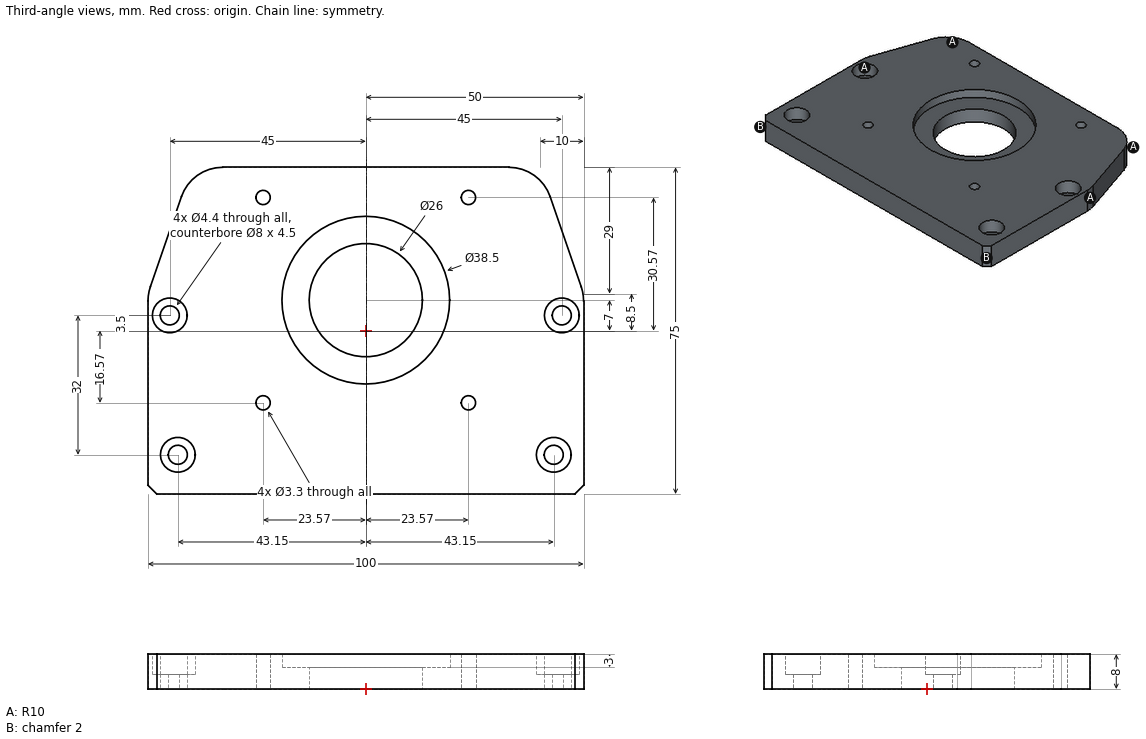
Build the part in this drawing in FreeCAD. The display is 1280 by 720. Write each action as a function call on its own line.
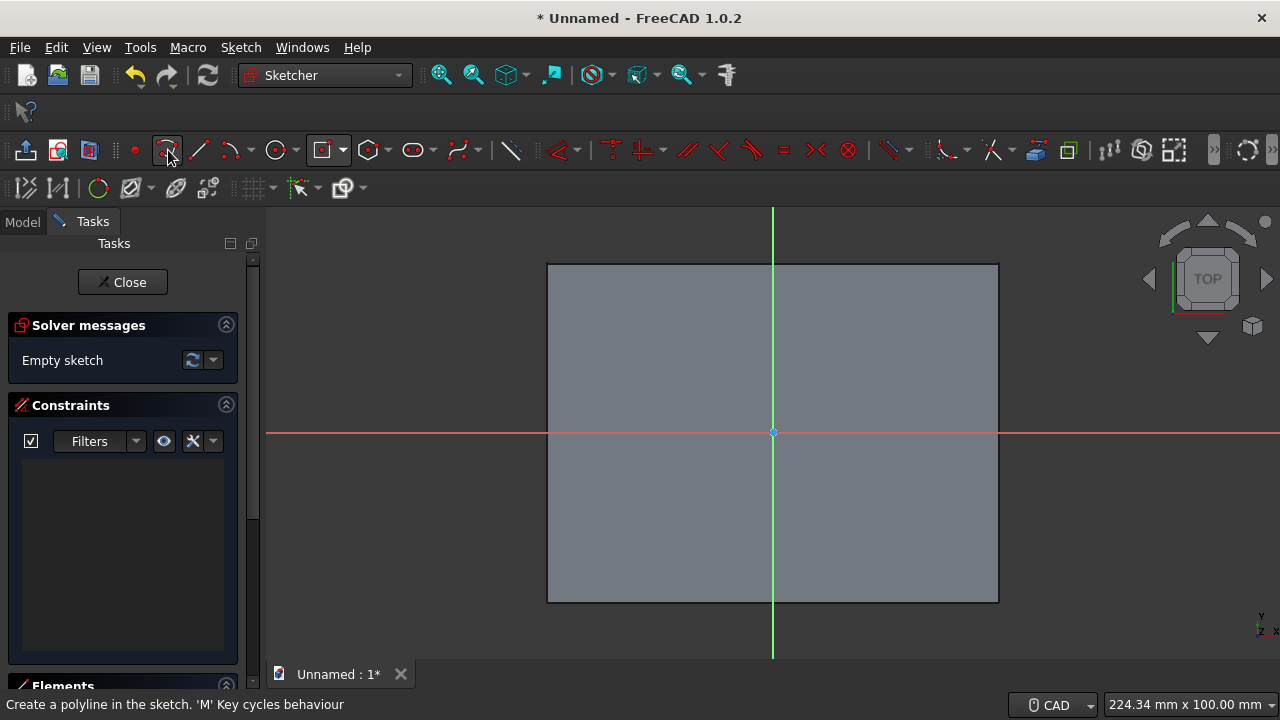
click(999, 395)
click(954, 264)
click(999, 264)
click(999, 396)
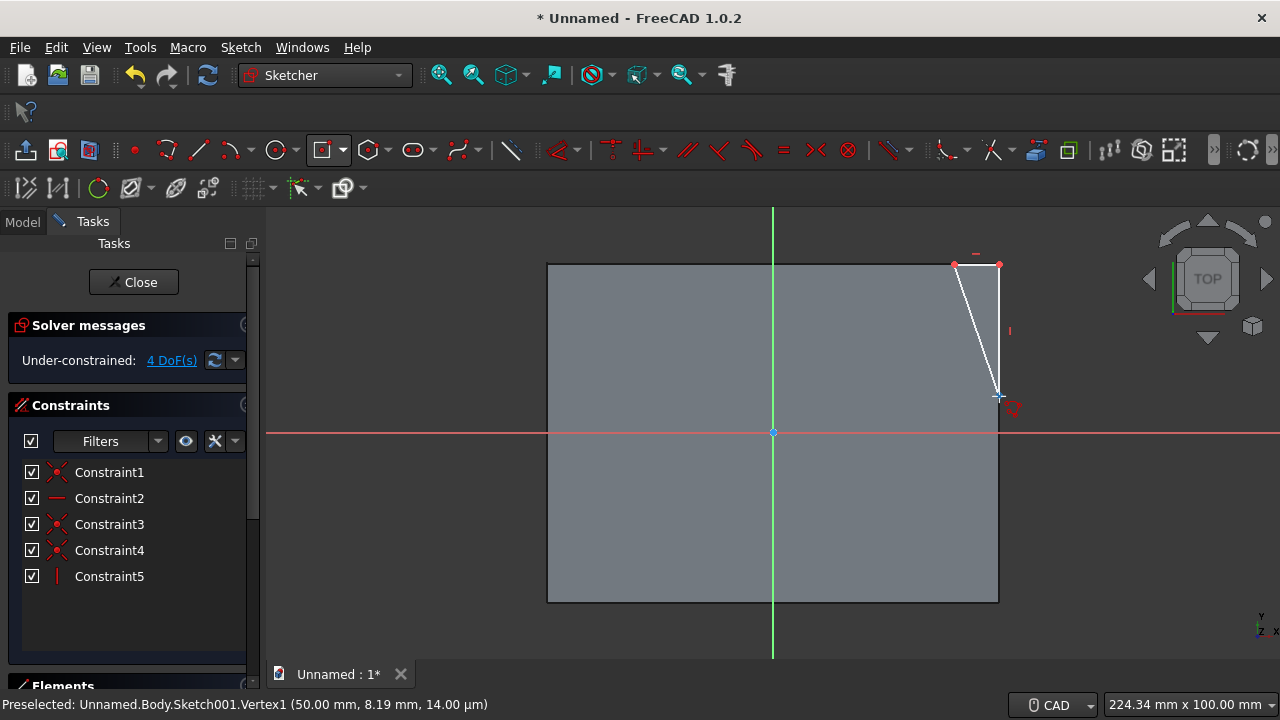
click(547, 395)
click(547, 264)
click(592, 264)
click(547, 396)
key(Escape)
key(Escape)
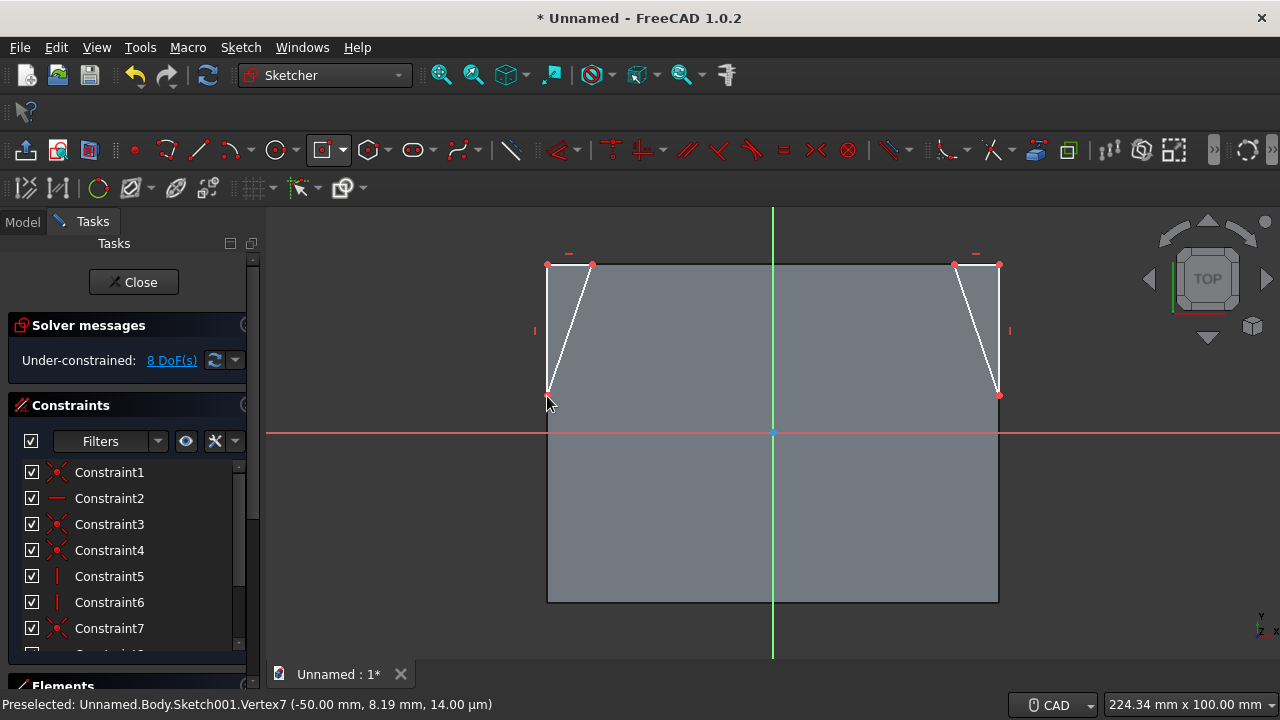
click(999, 396)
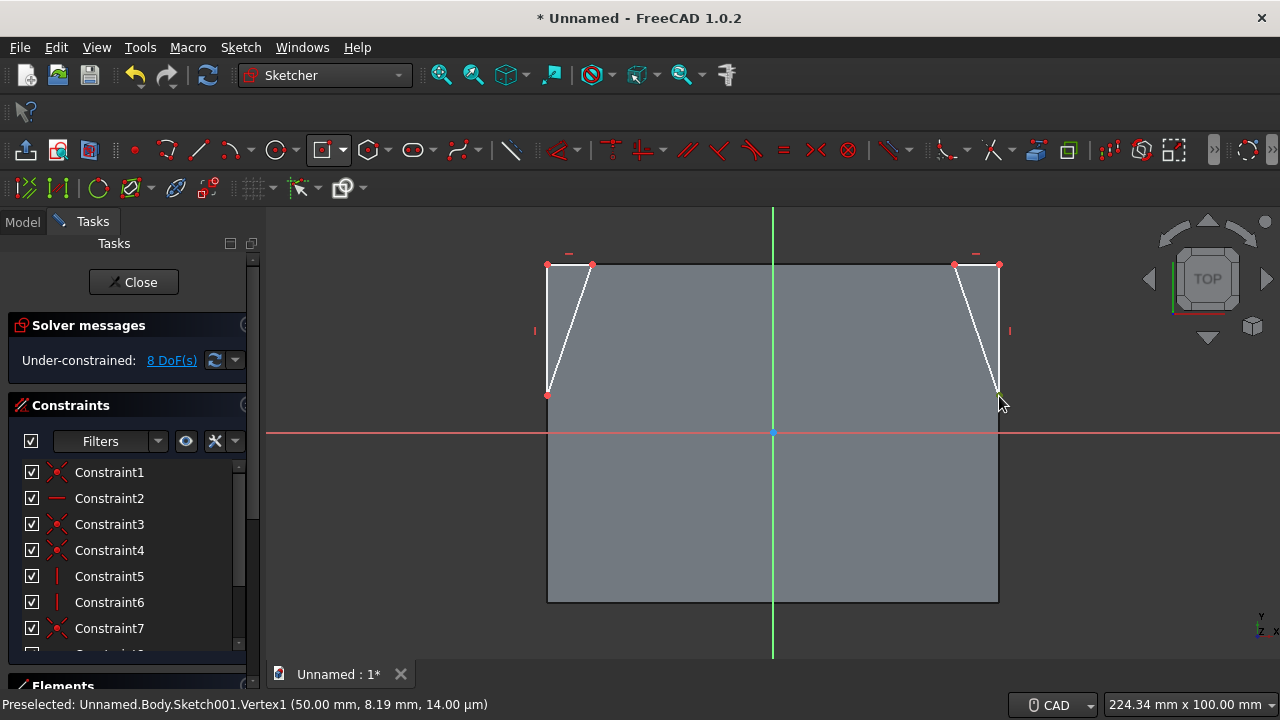
click(547, 396)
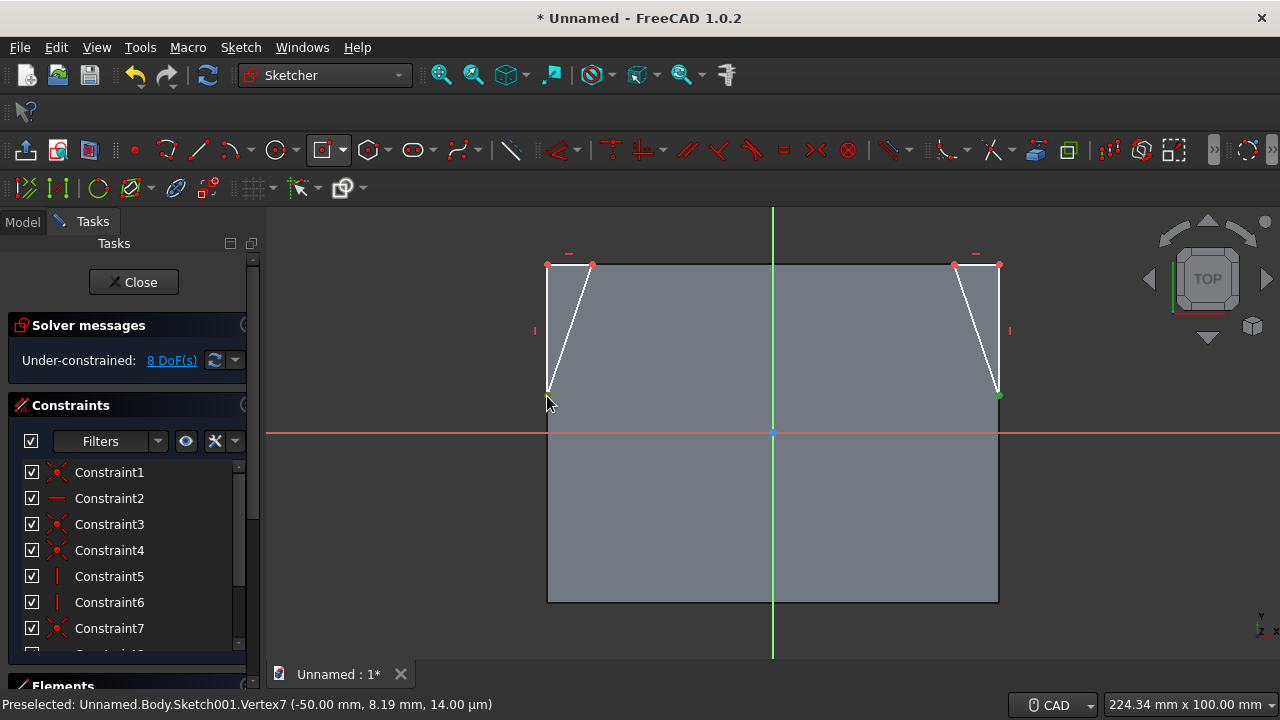
click(773, 603)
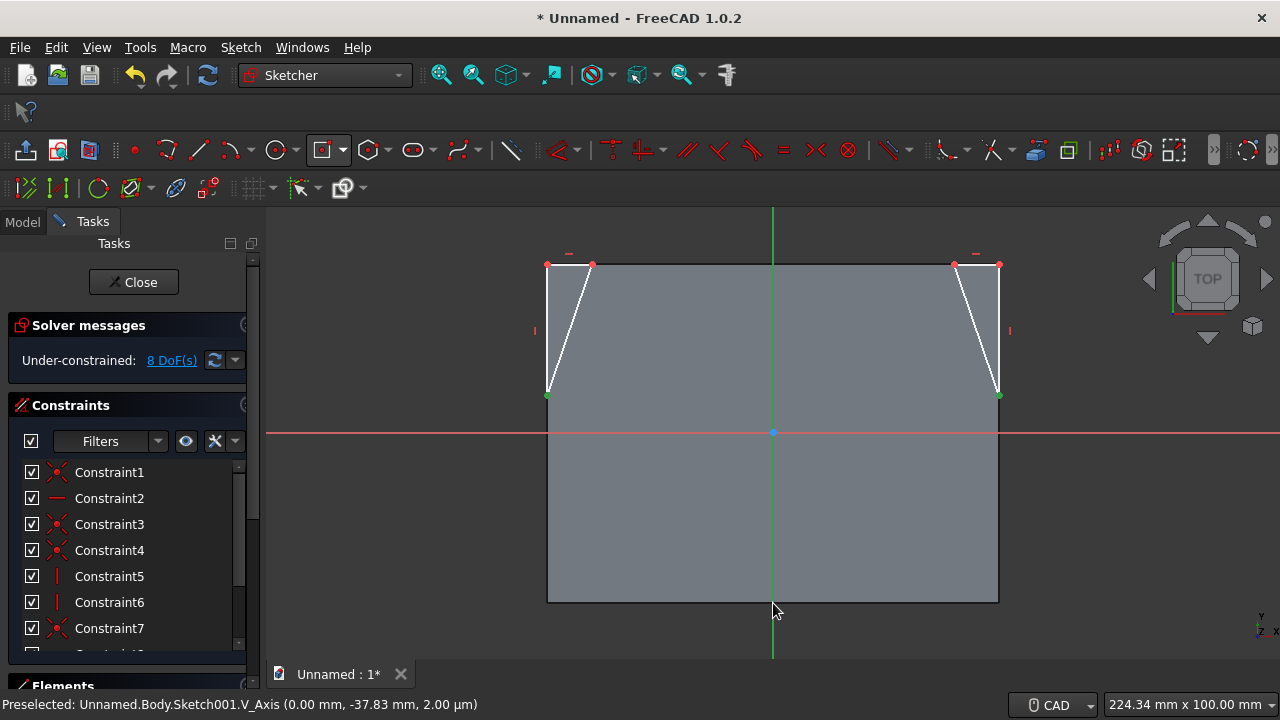
click(816, 150)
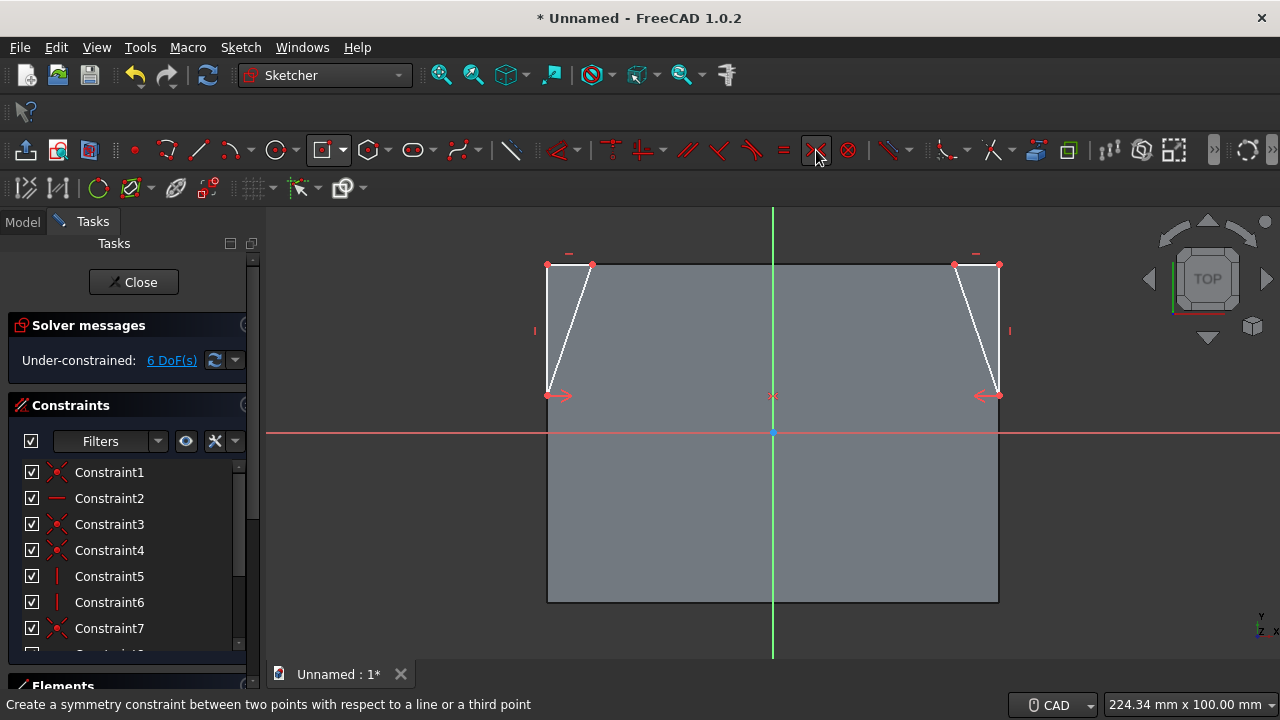
click(954, 265)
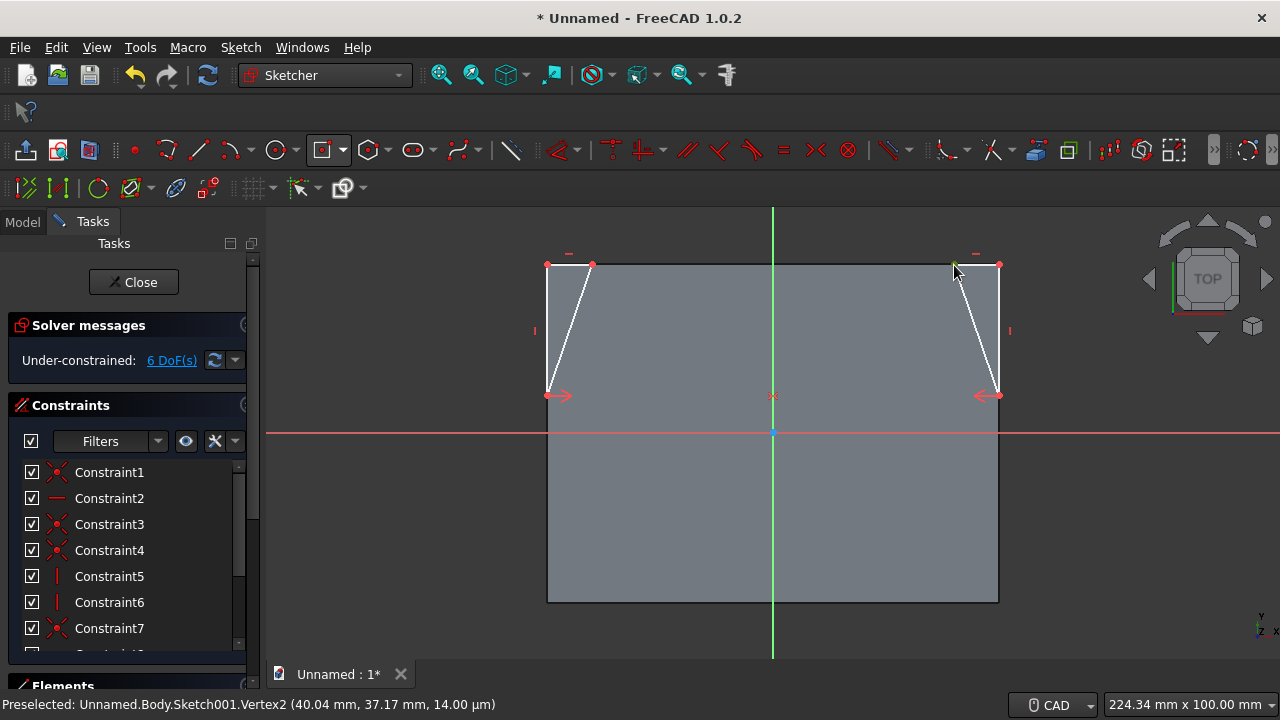
click(592, 265)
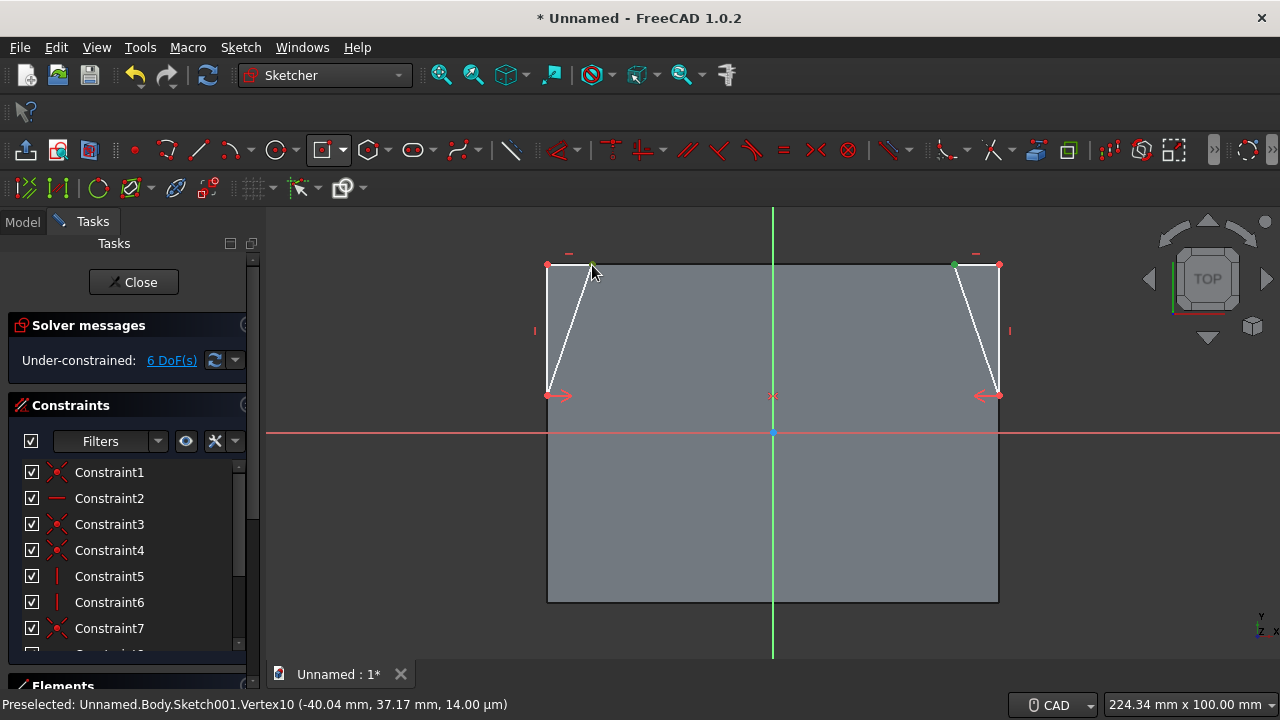
click(773, 603)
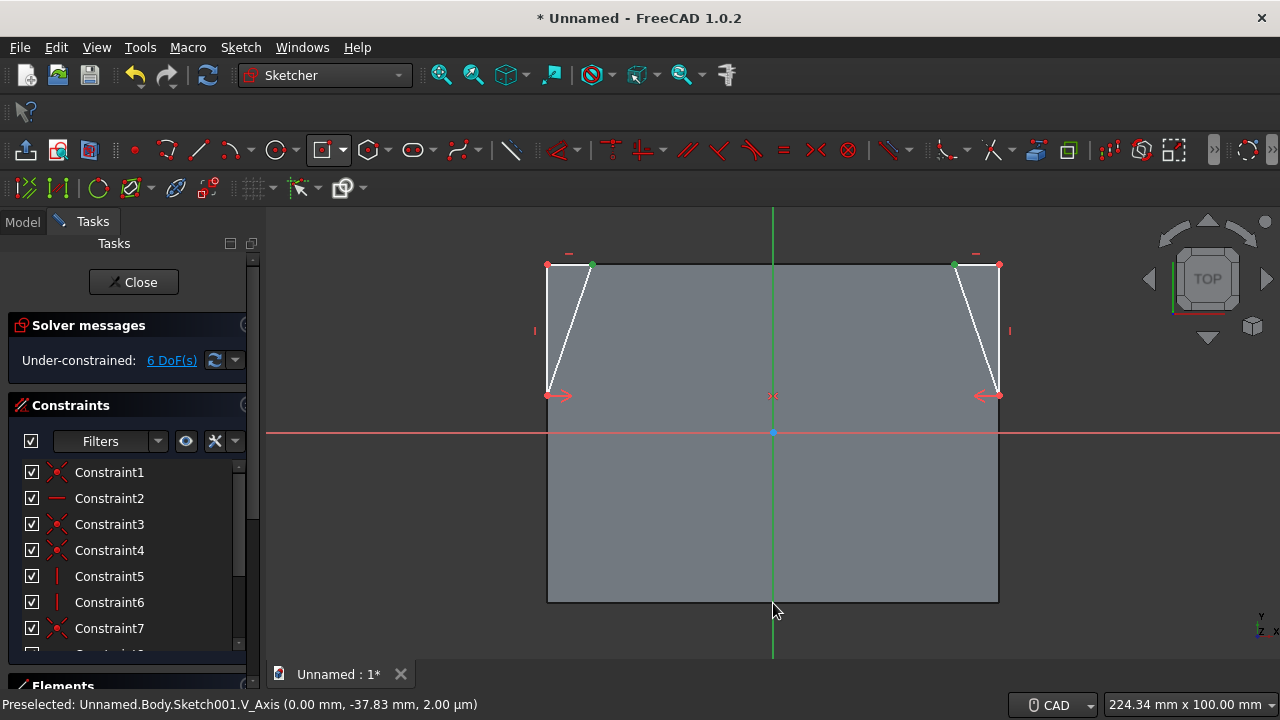
click(816, 150)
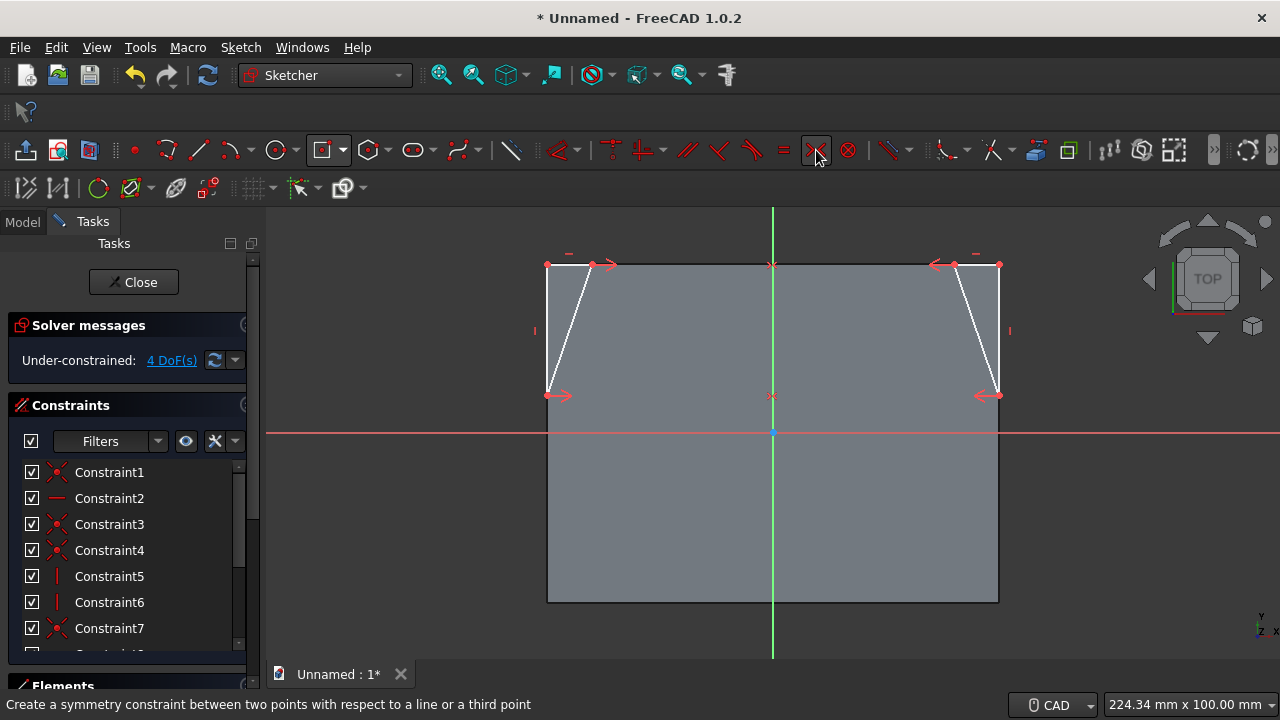
click(967, 265)